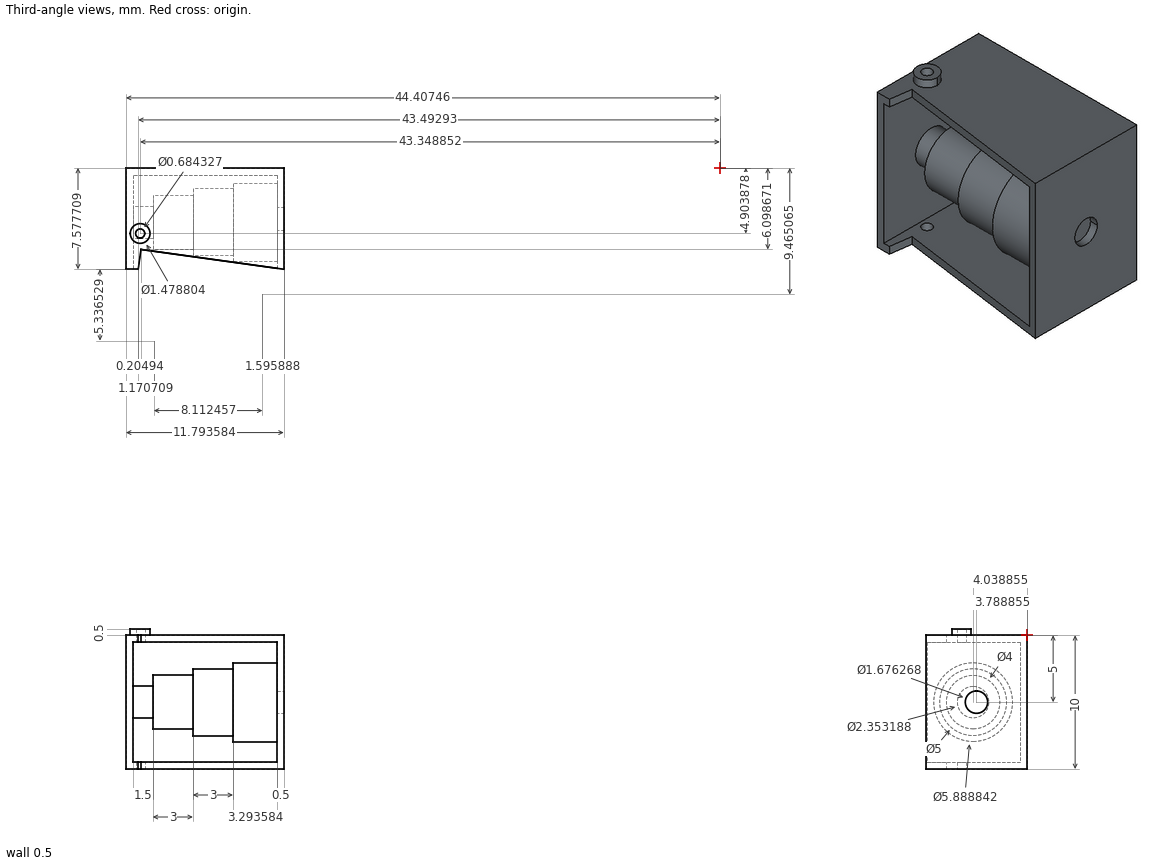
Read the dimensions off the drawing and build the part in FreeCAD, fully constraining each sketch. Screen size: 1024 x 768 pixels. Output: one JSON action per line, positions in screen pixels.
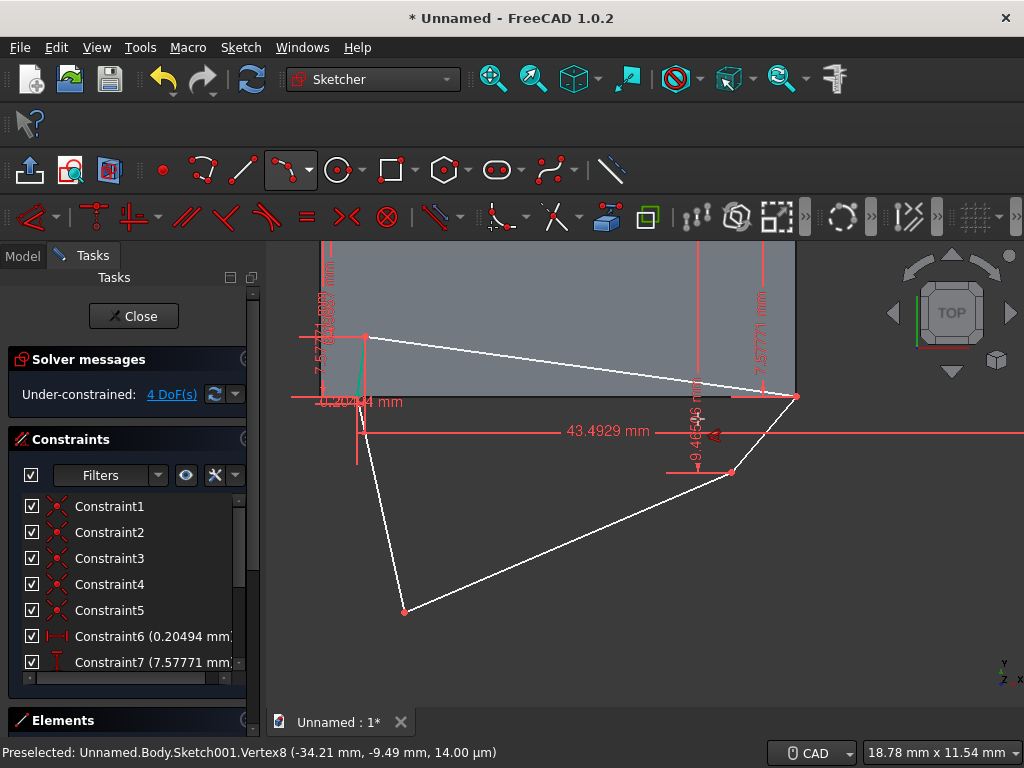
{"action": "left_click", "coordinate": [371, 461]}
{"action": "left_click", "coordinate": [381, 647]}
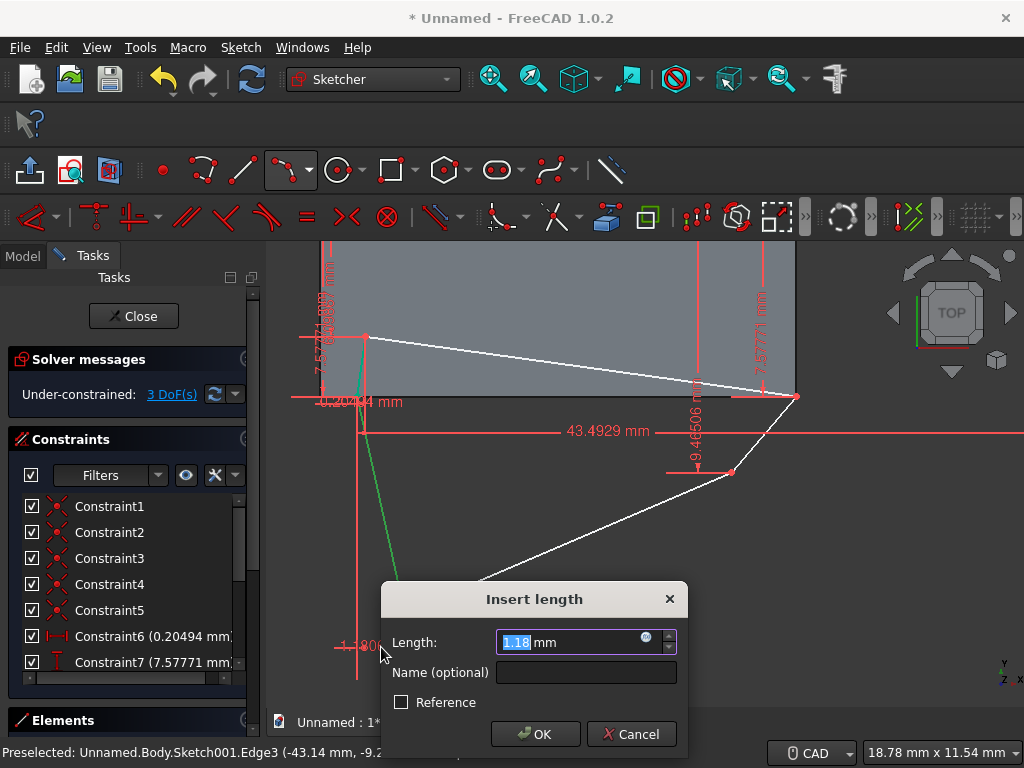
{"action": "type", "text": "1.170709"}
{"action": "key", "text": "Return"}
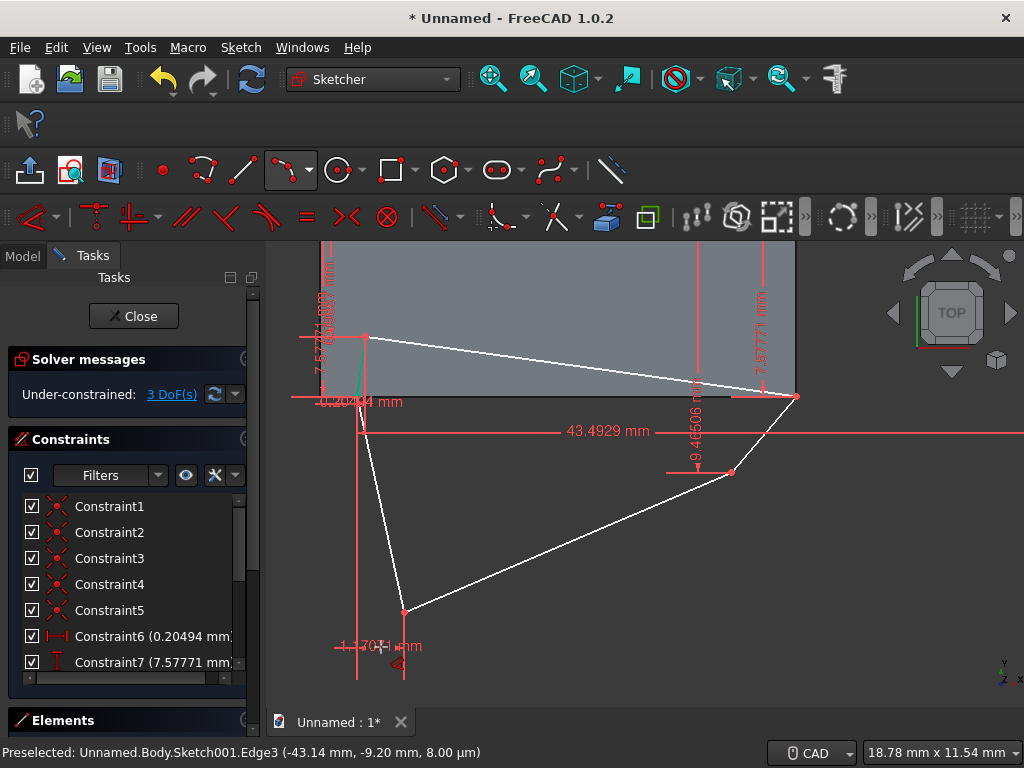
{"action": "left_click", "coordinate": [371, 461]}
{"action": "left_click", "coordinate": [323, 505]}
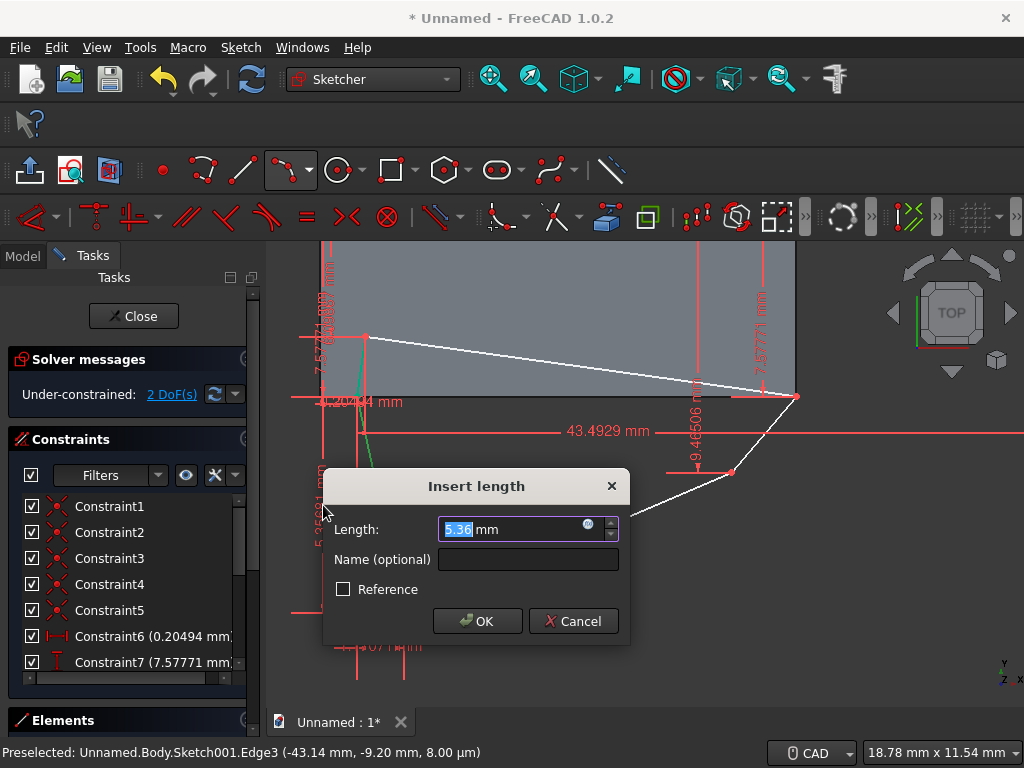
{"action": "type", "text": "5.336529"}
{"action": "key", "text": "Return"}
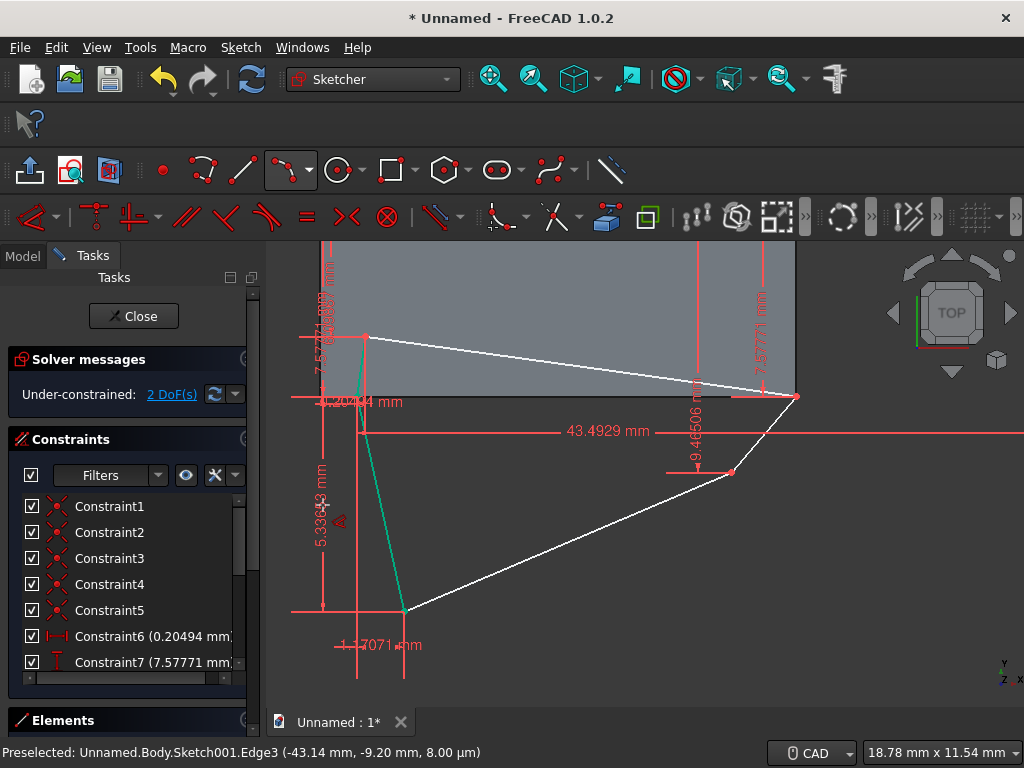
{"action": "left_click", "coordinate": [503, 570]}
{"action": "left_click", "coordinate": [568, 646]}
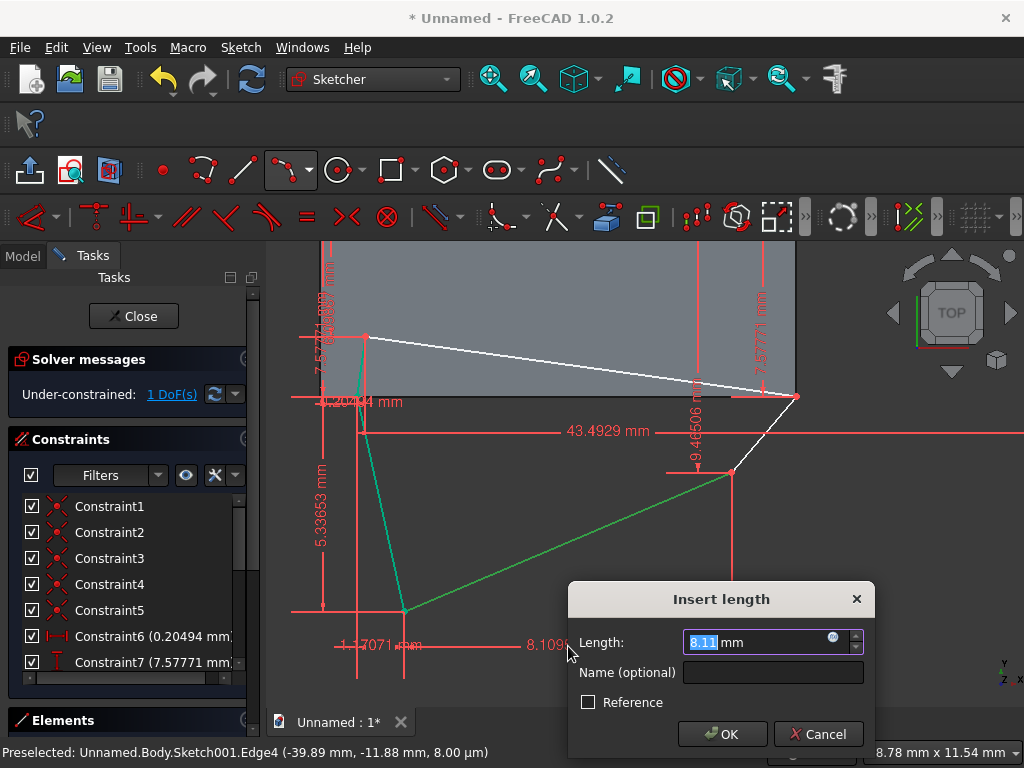
{"action": "type", "text": "8.112457"}
{"action": "key", "text": "Return"}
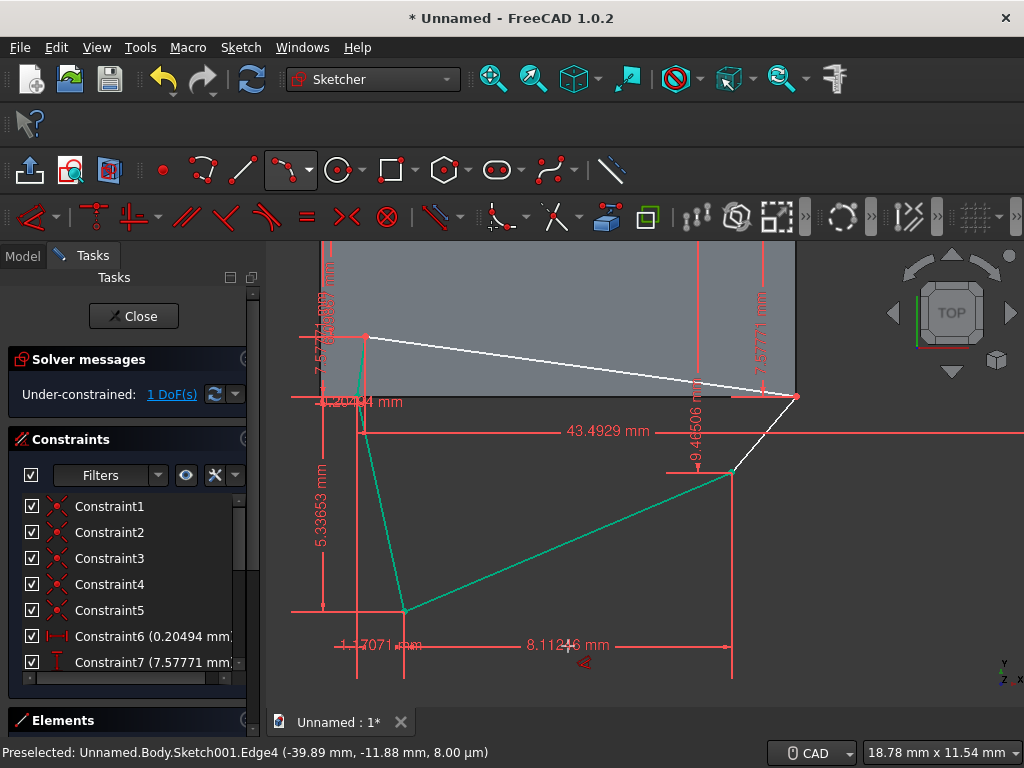
{"action": "left_click", "coordinate": [751, 450]}
{"action": "left_click", "coordinate": [764, 363]}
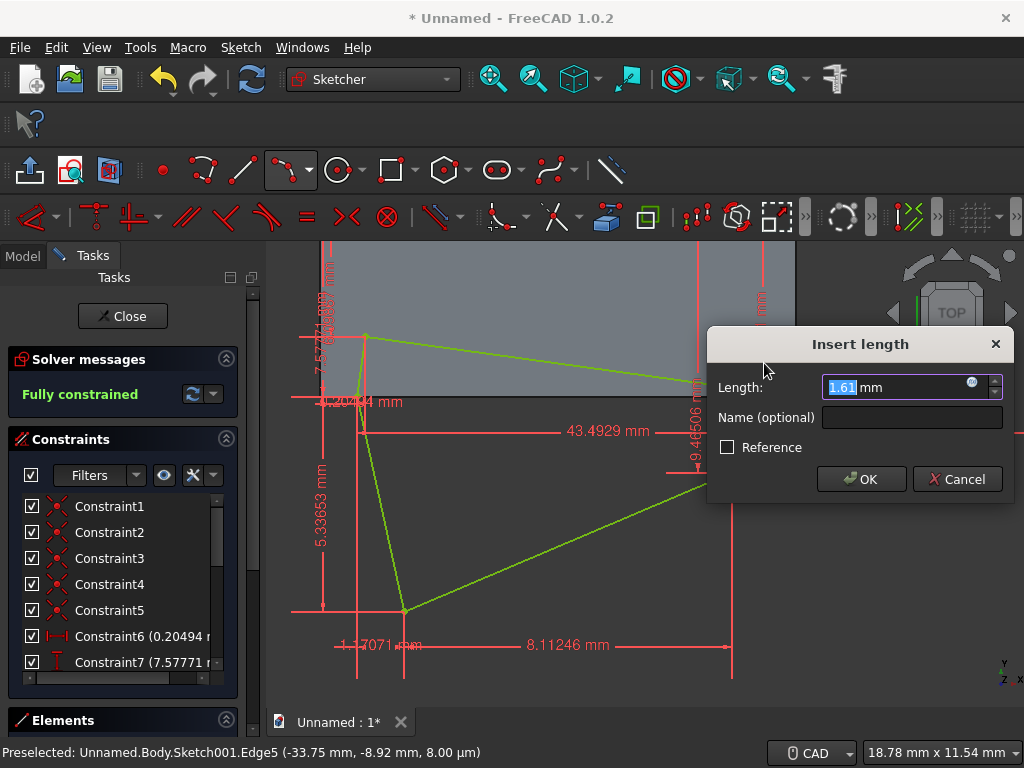
{"action": "type", "text": "1.595888"}
{"action": "key", "text": "Return"}
{"action": "key", "text": "Escape"}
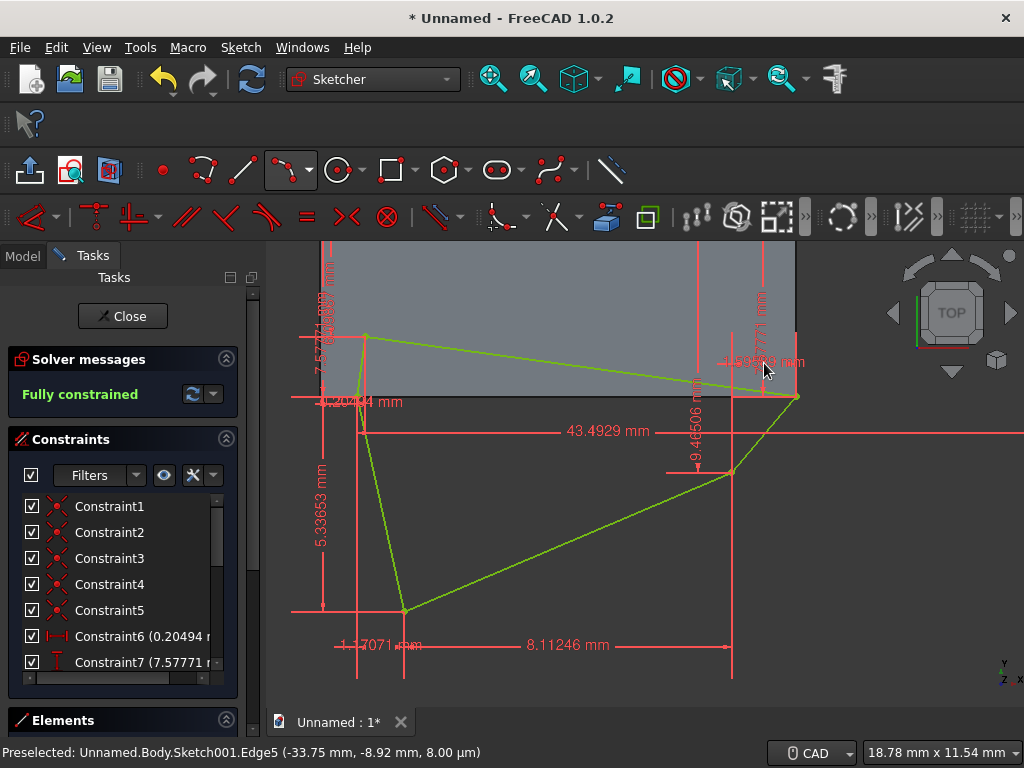
{"action": "left_click", "coordinate": [123, 316]}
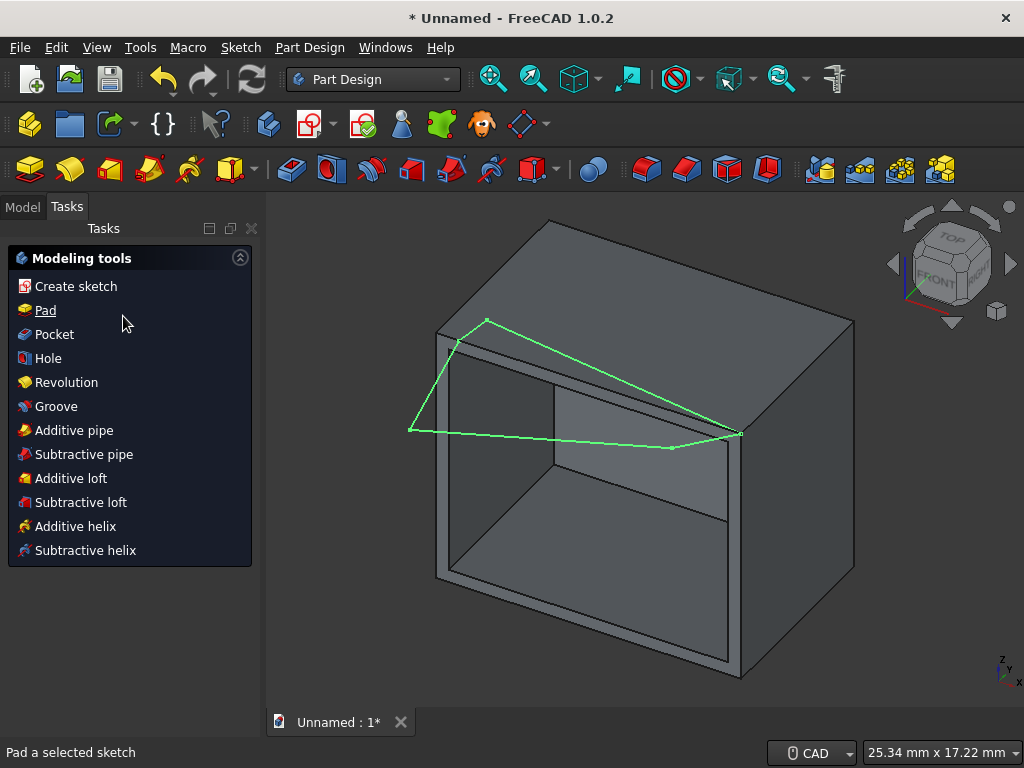
{"action": "left_click", "coordinate": [292, 170]}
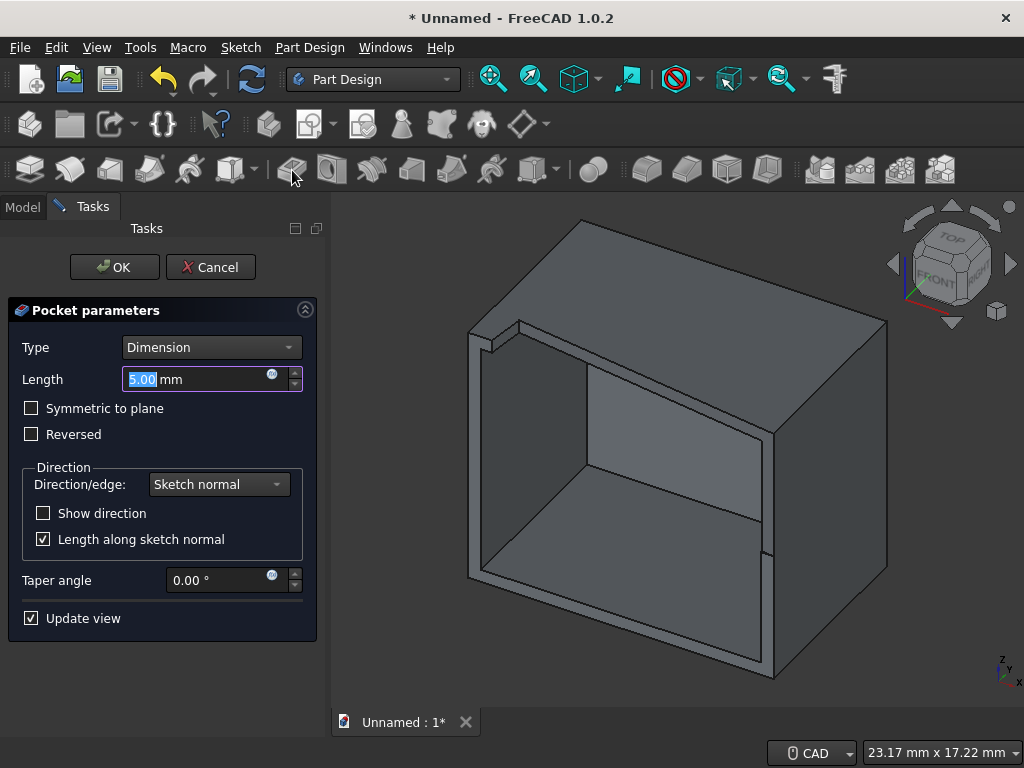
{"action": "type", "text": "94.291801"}
{"action": "key", "text": "Tab"}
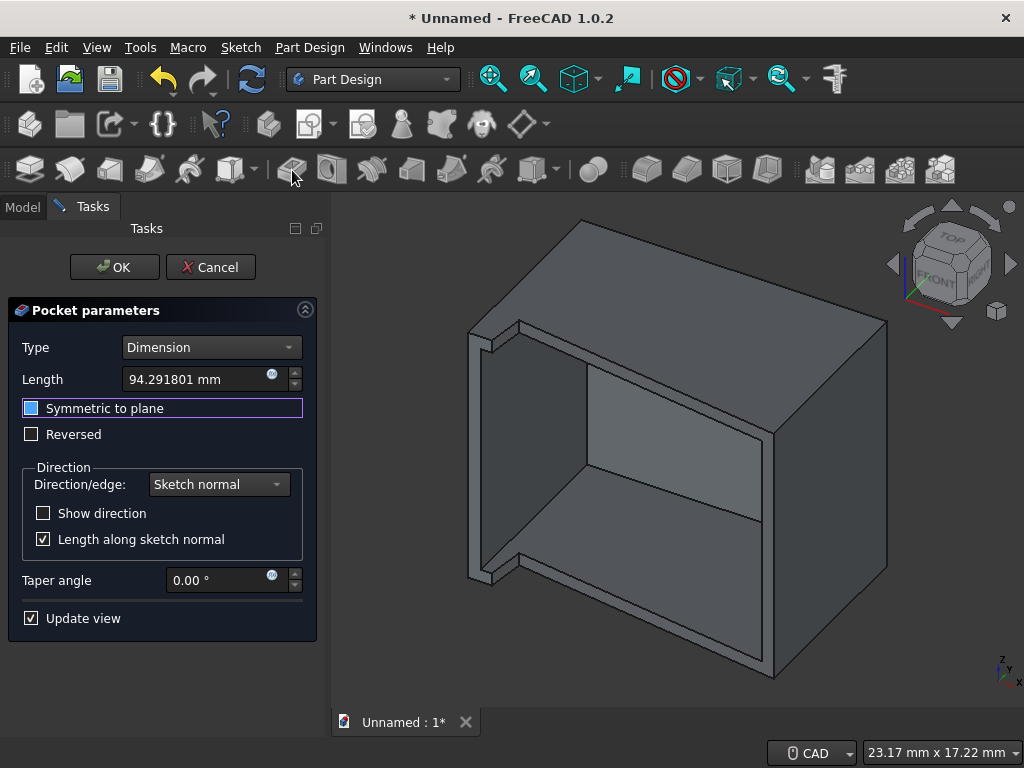
{"action": "left_click", "coordinate": [30, 408]}